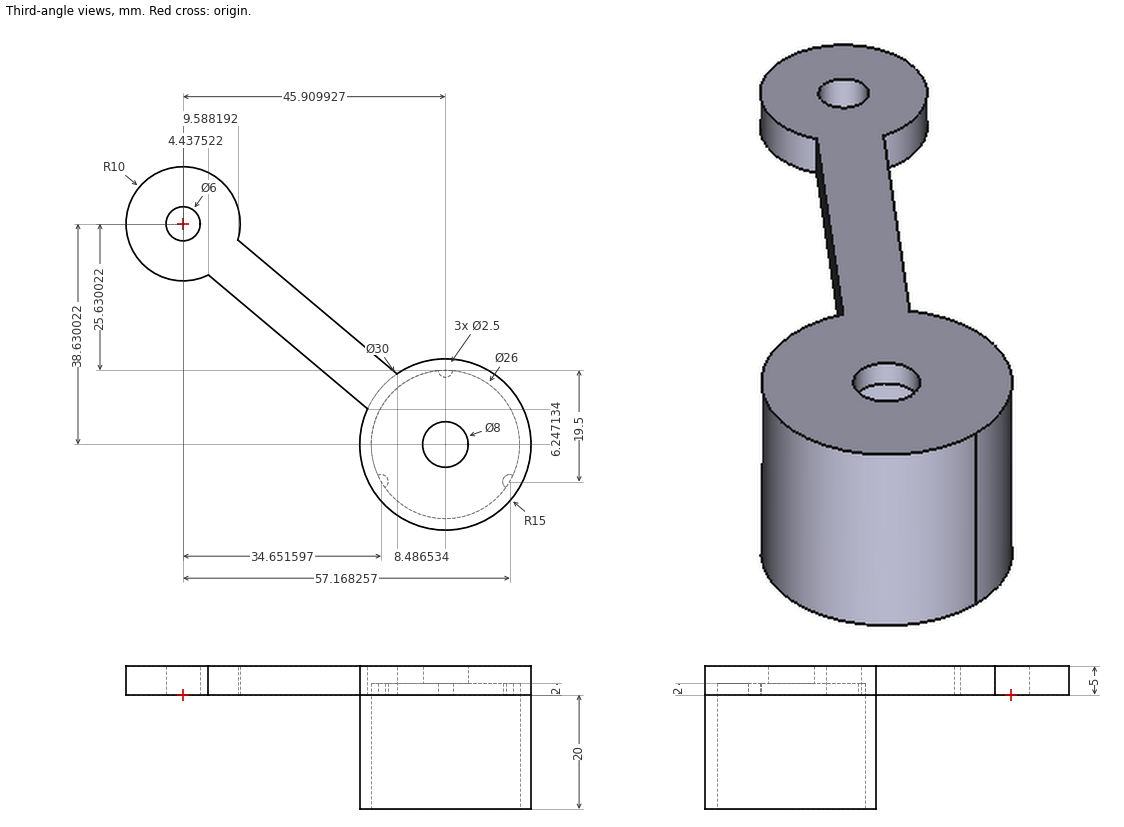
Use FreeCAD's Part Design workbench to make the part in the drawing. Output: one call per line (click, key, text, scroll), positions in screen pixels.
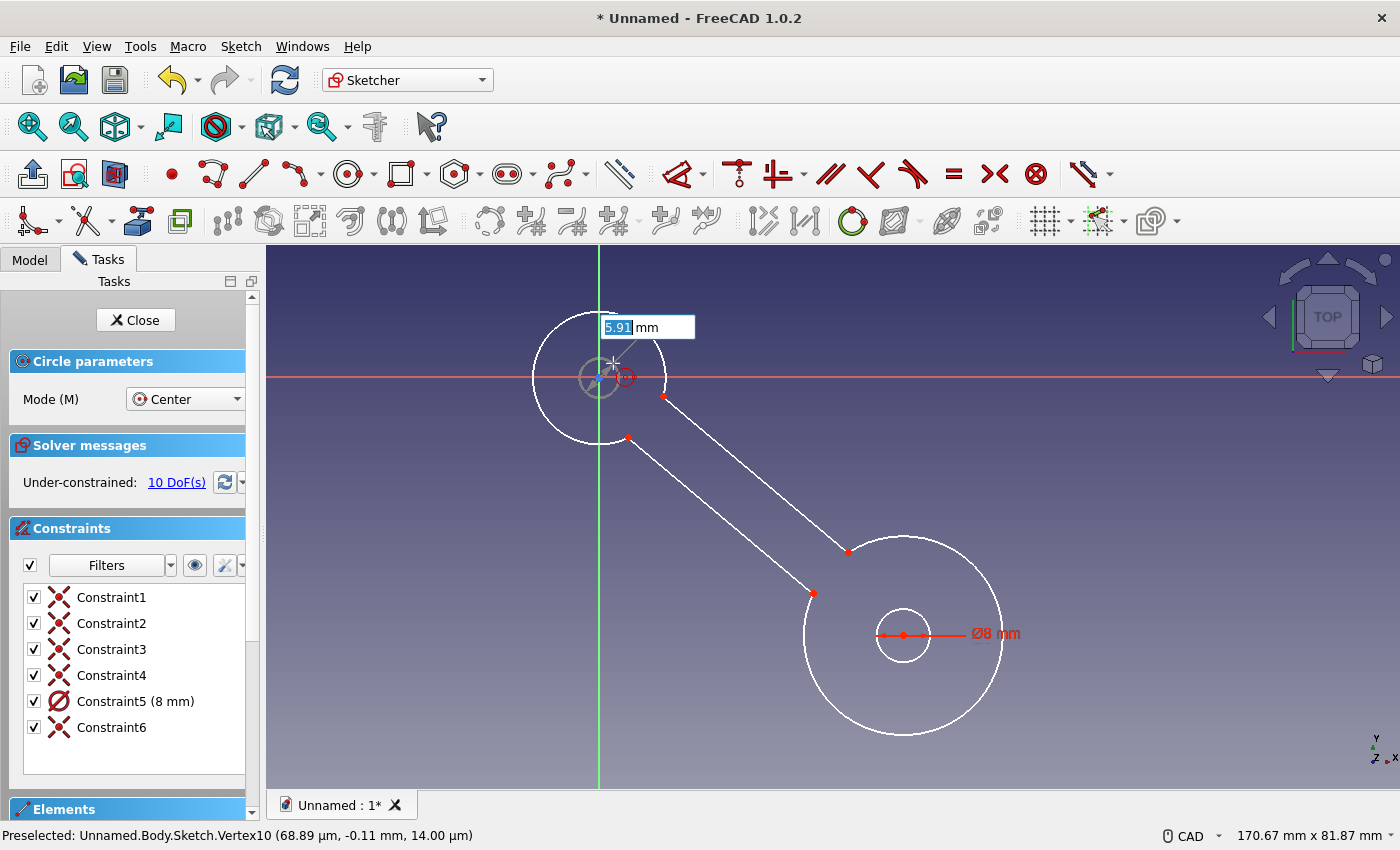
text(6)
key(Return)
key(Escape)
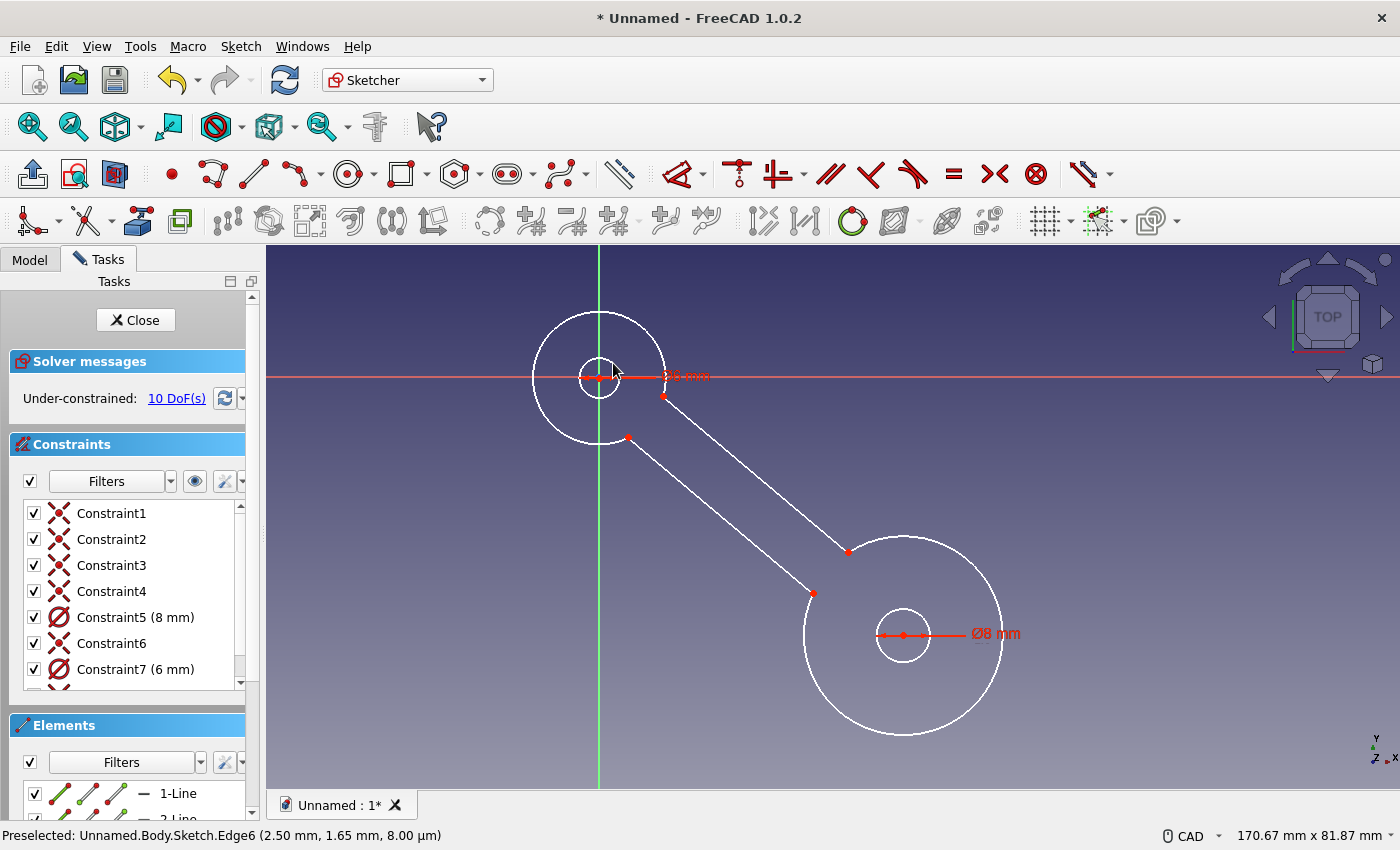
scroll(599, 378, up, 4)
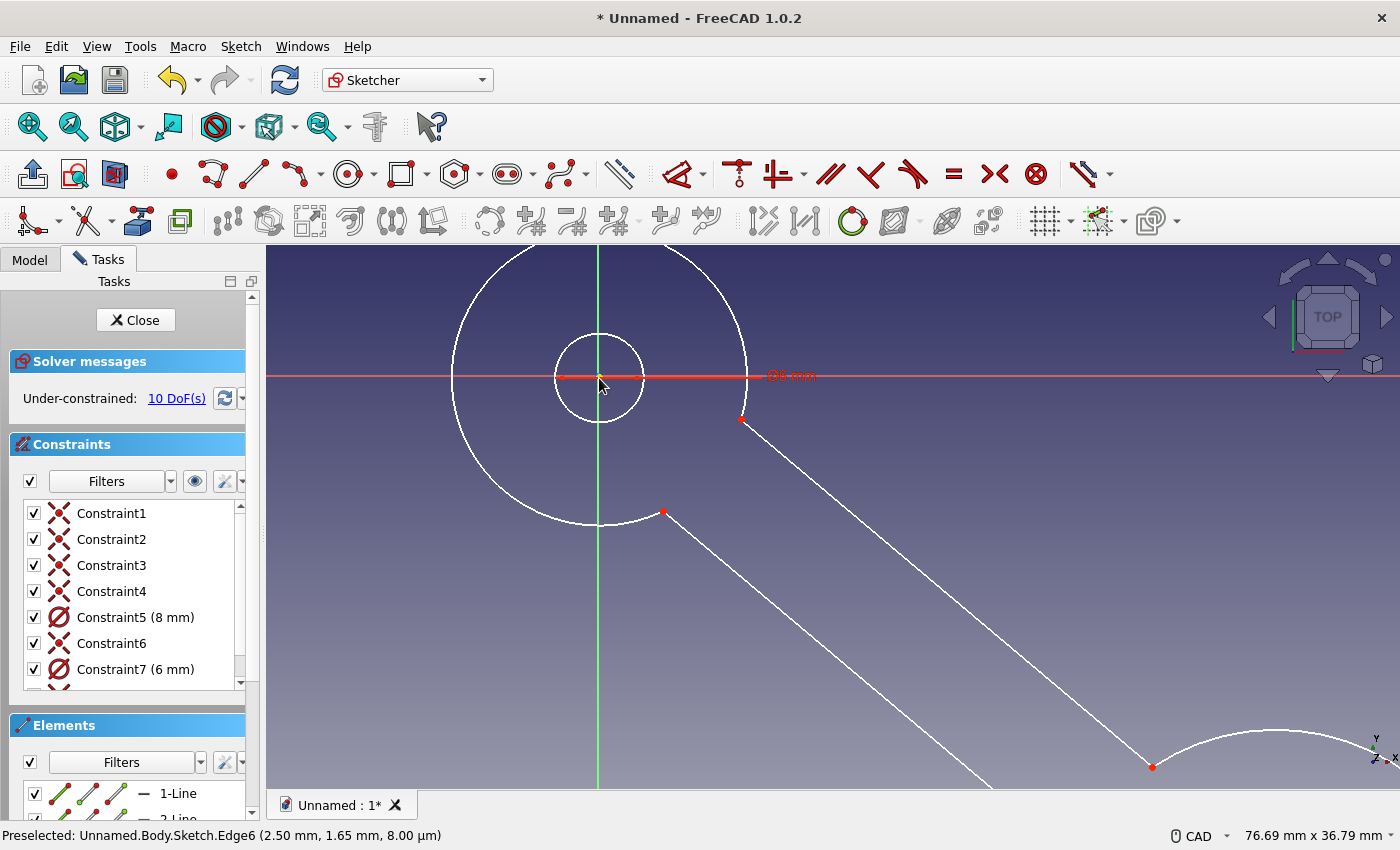
drag(588, 366, 609, 388)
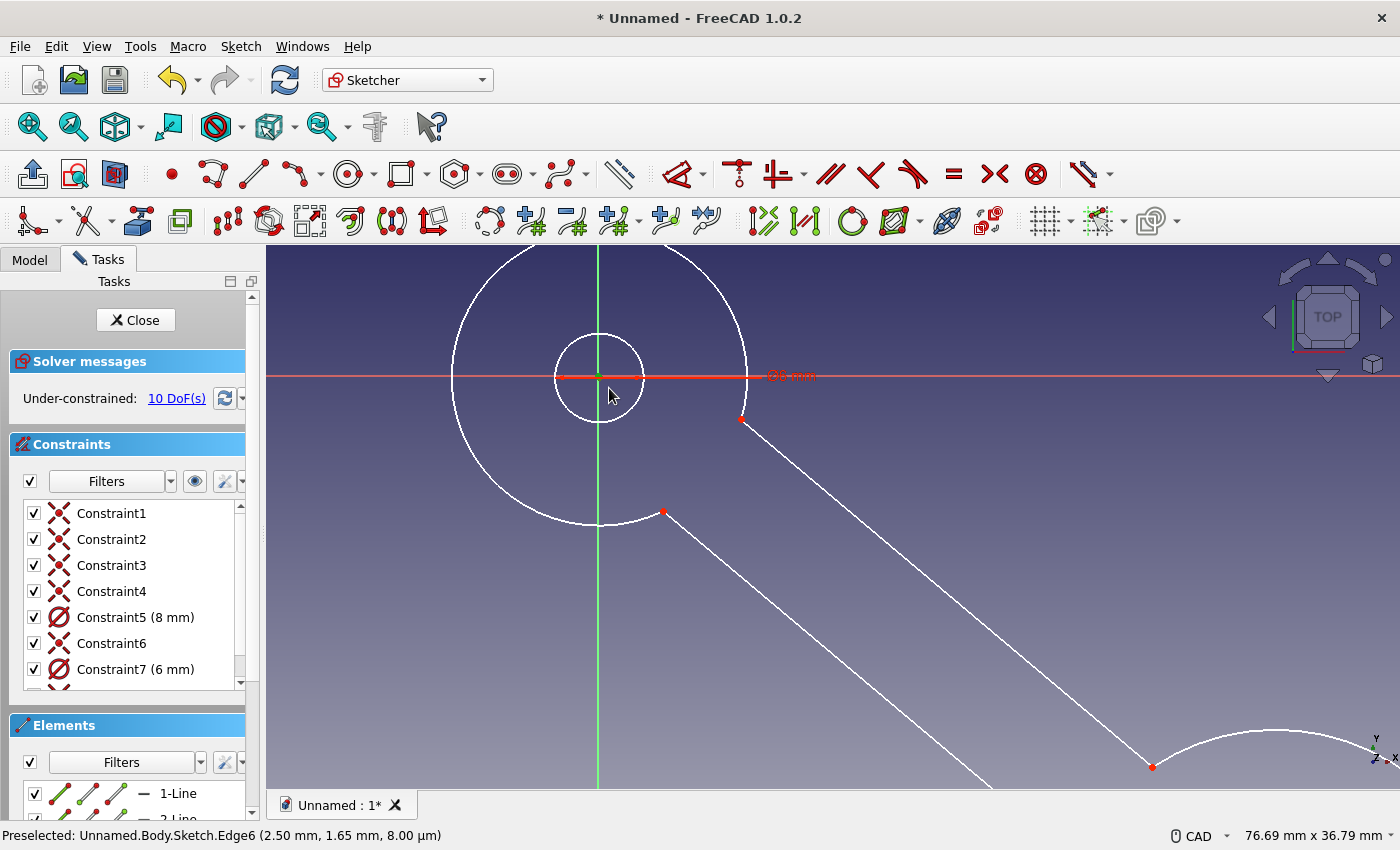
click(737, 174)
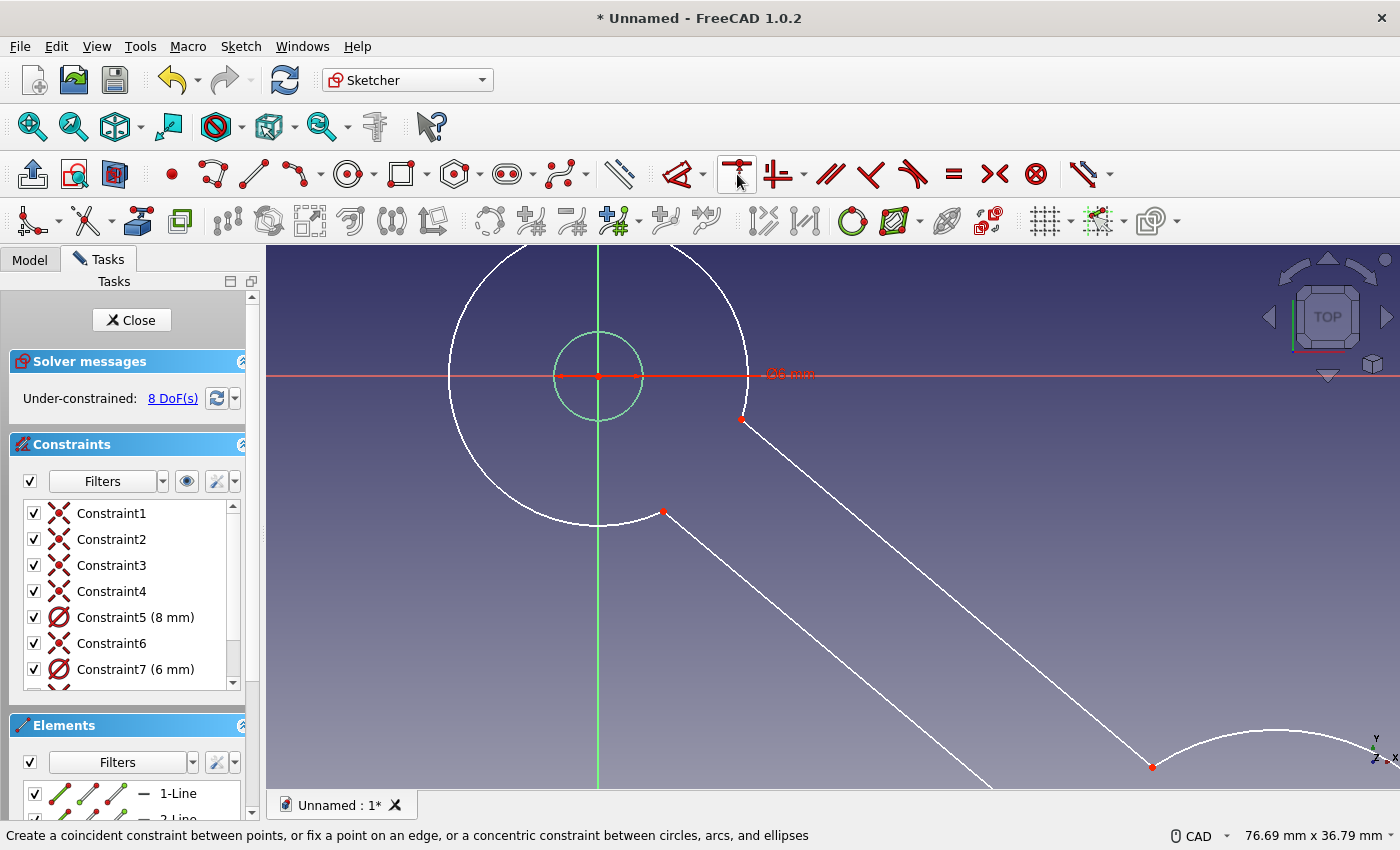
click(676, 174)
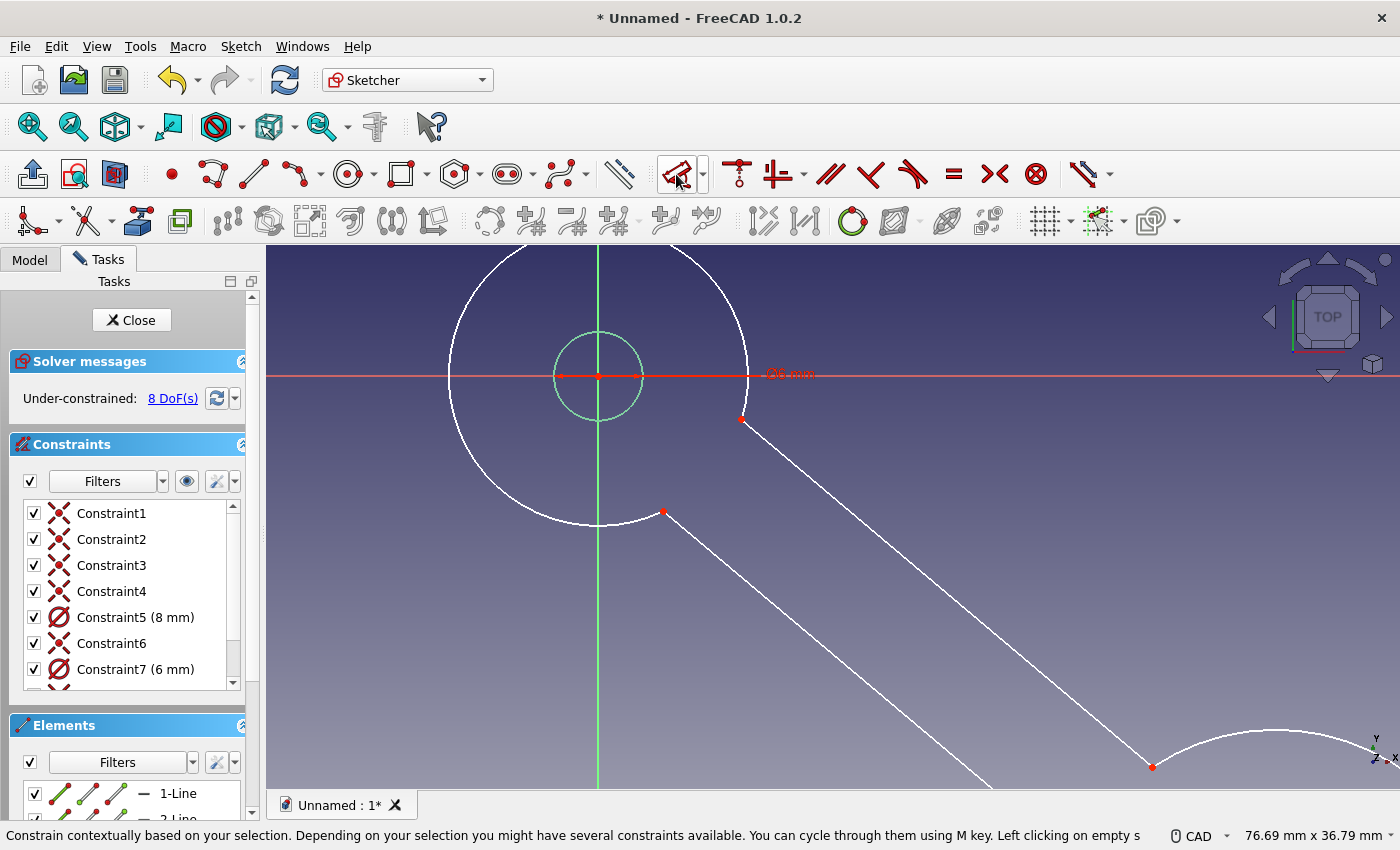
scroll(600, 379, down, 4)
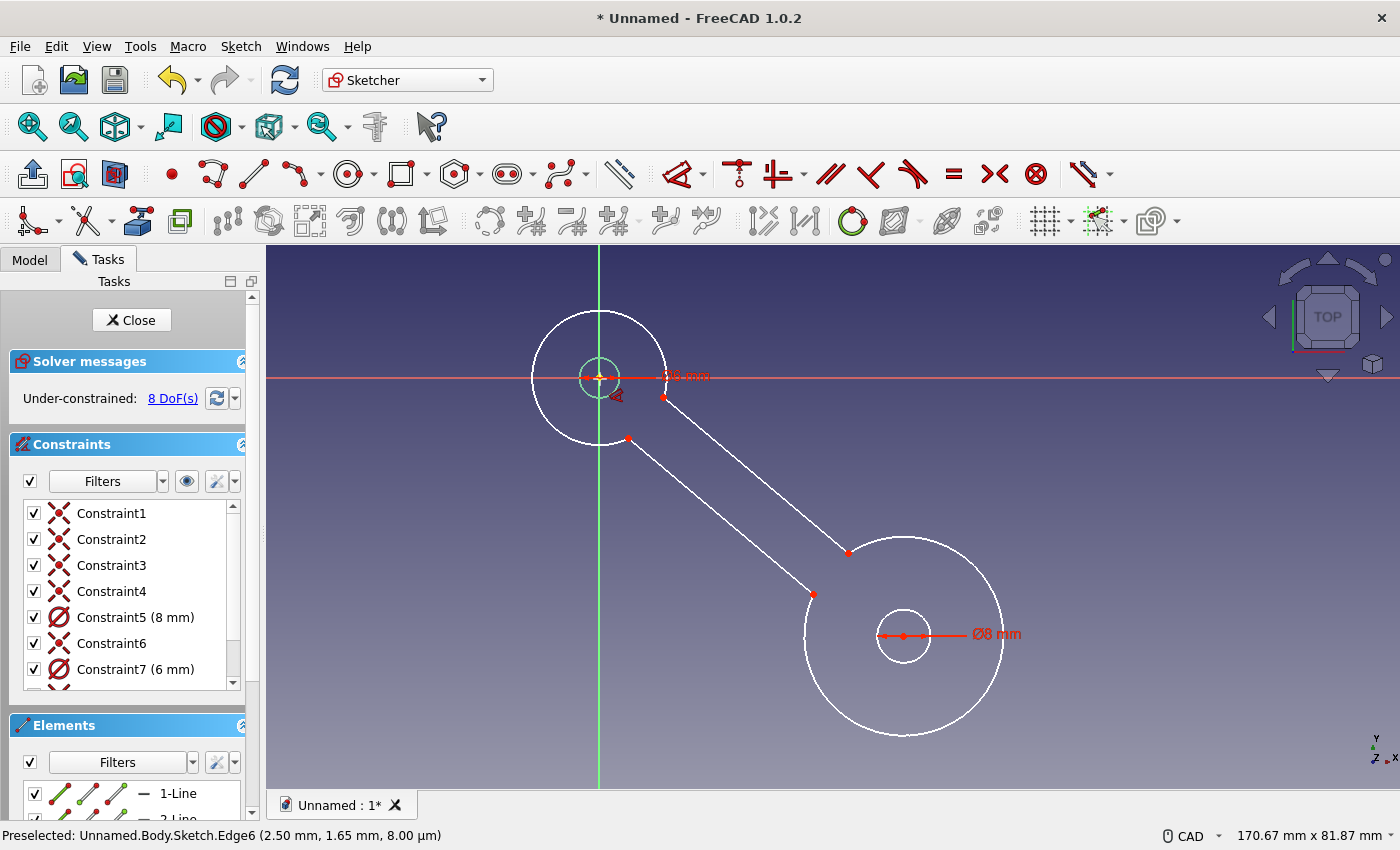
click(876, 732)
click(811, 730)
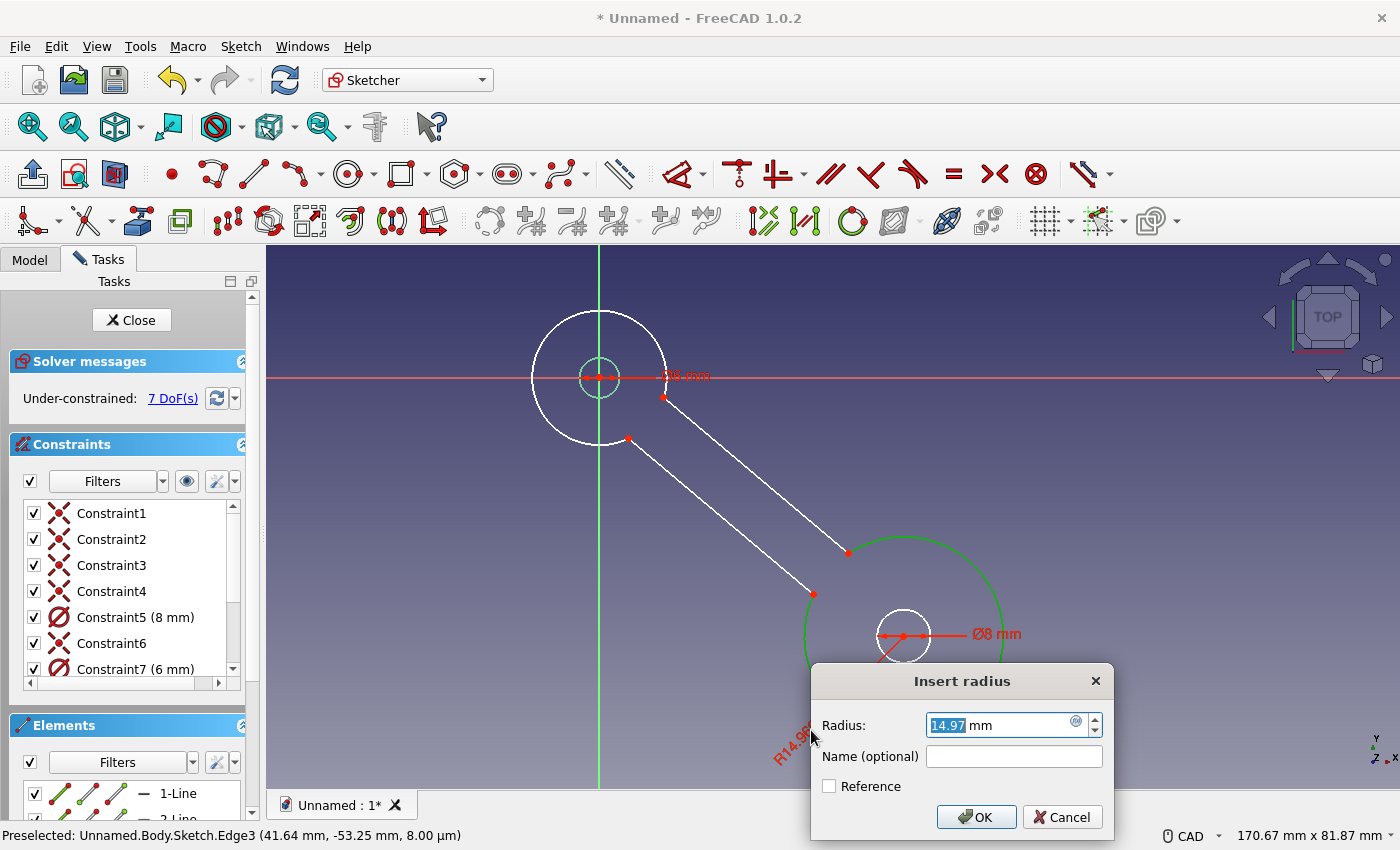
text(15)
key(Return)